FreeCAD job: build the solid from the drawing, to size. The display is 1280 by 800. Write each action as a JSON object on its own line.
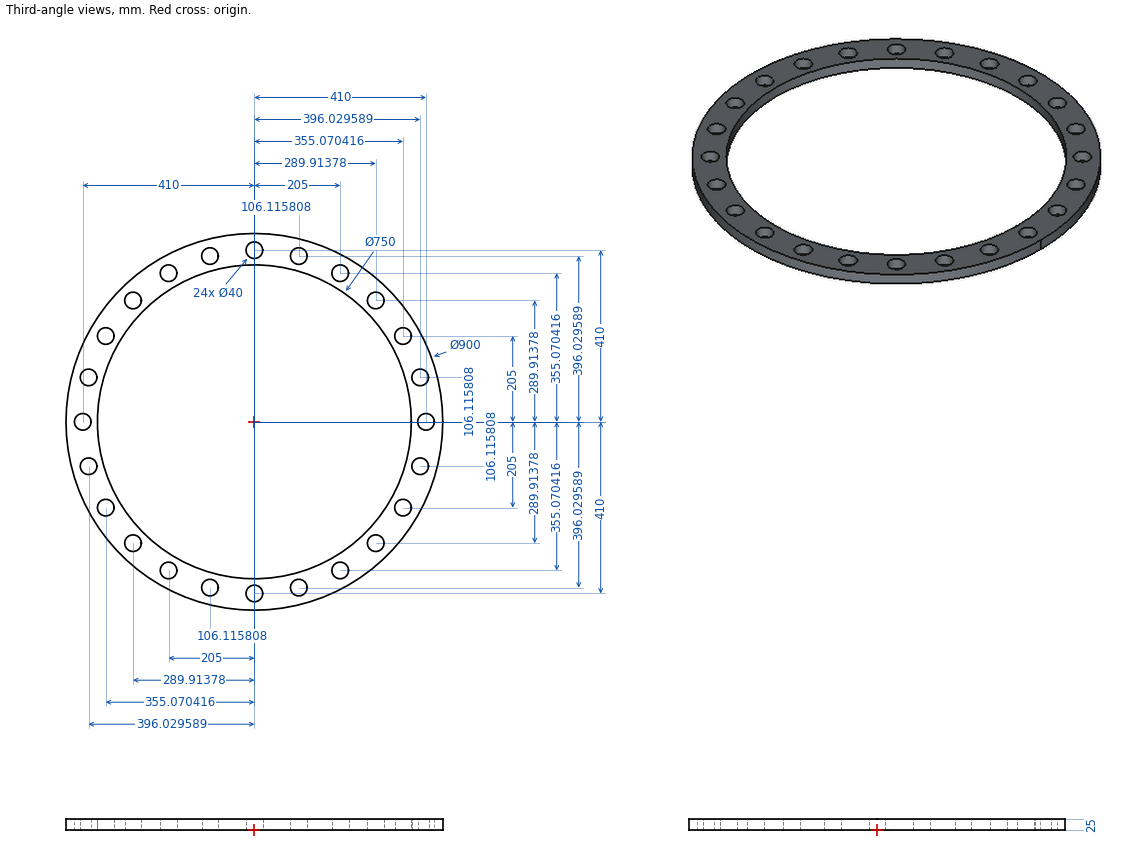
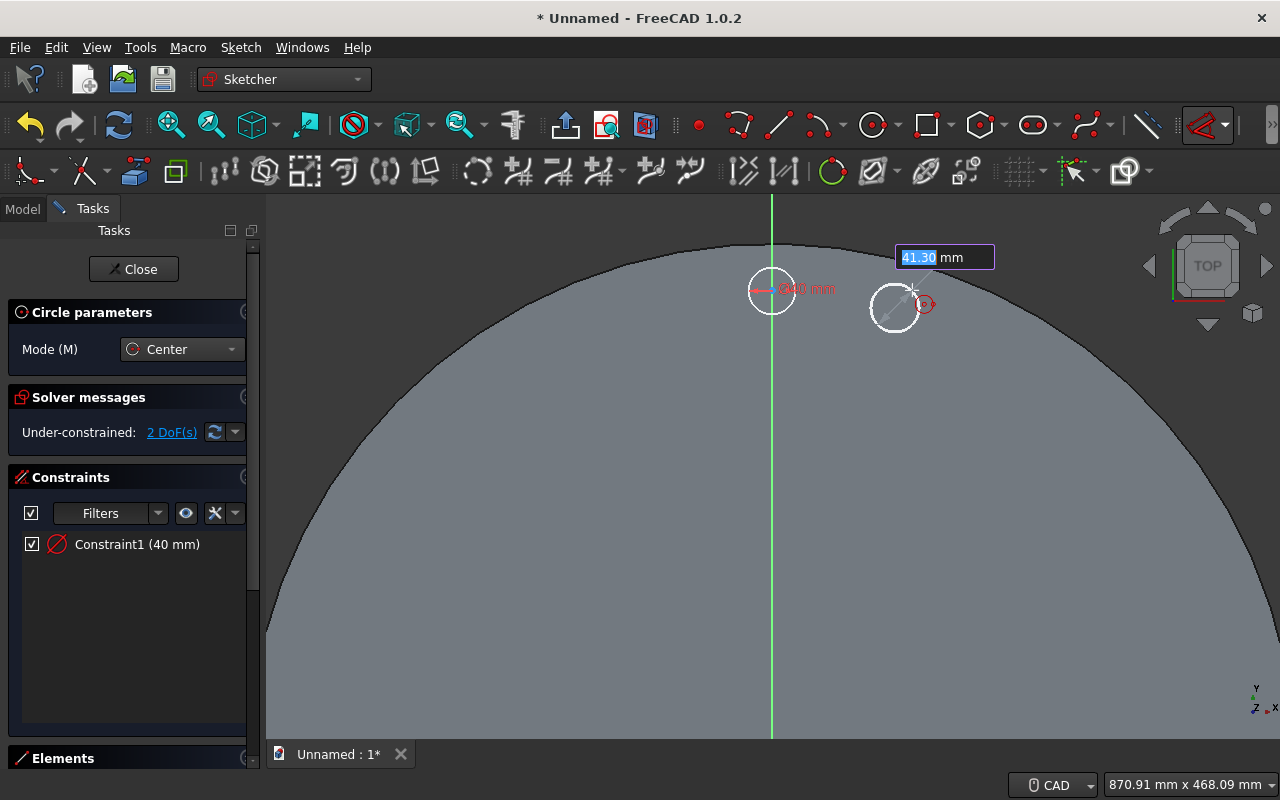
{"action": "type", "text": "40"}
{"action": "key", "text": "Return"}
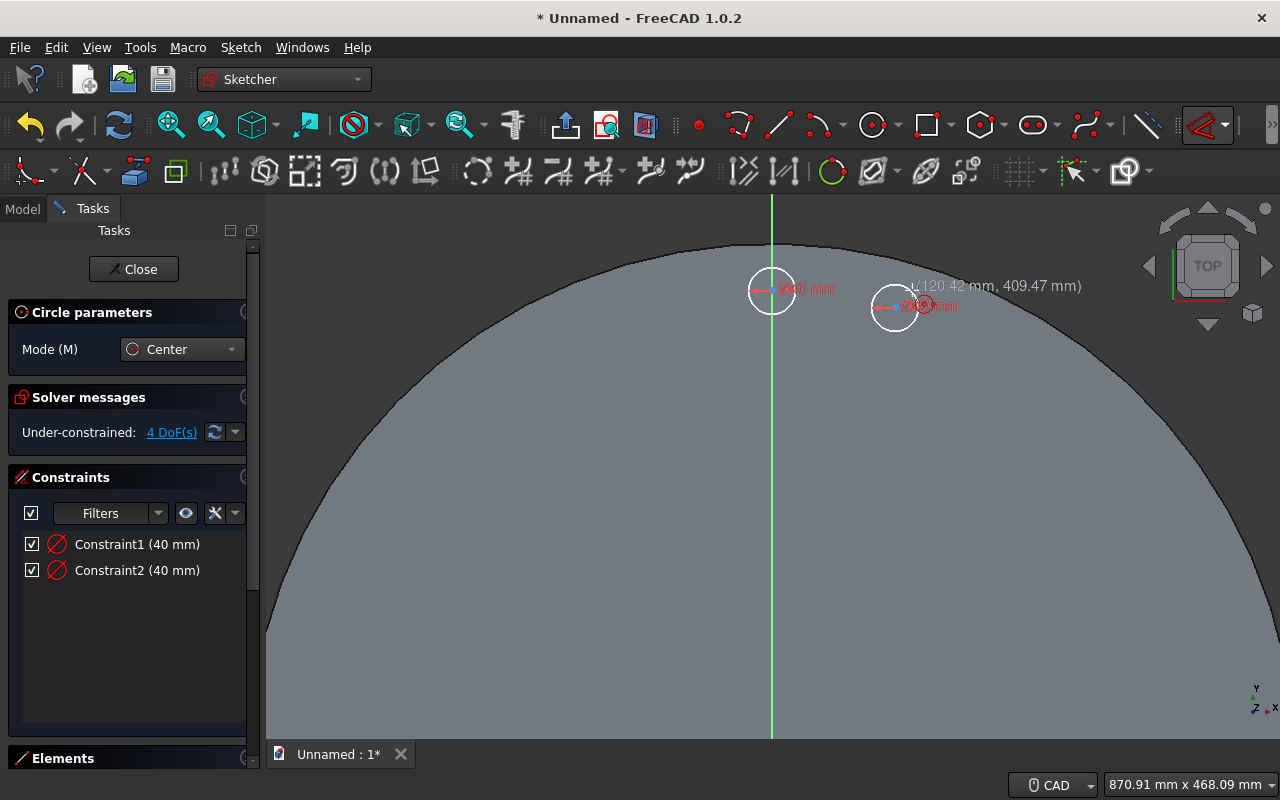
{"action": "left_click", "coordinate": [1010, 354]}
{"action": "mouse_move", "coordinate": [1027, 338]}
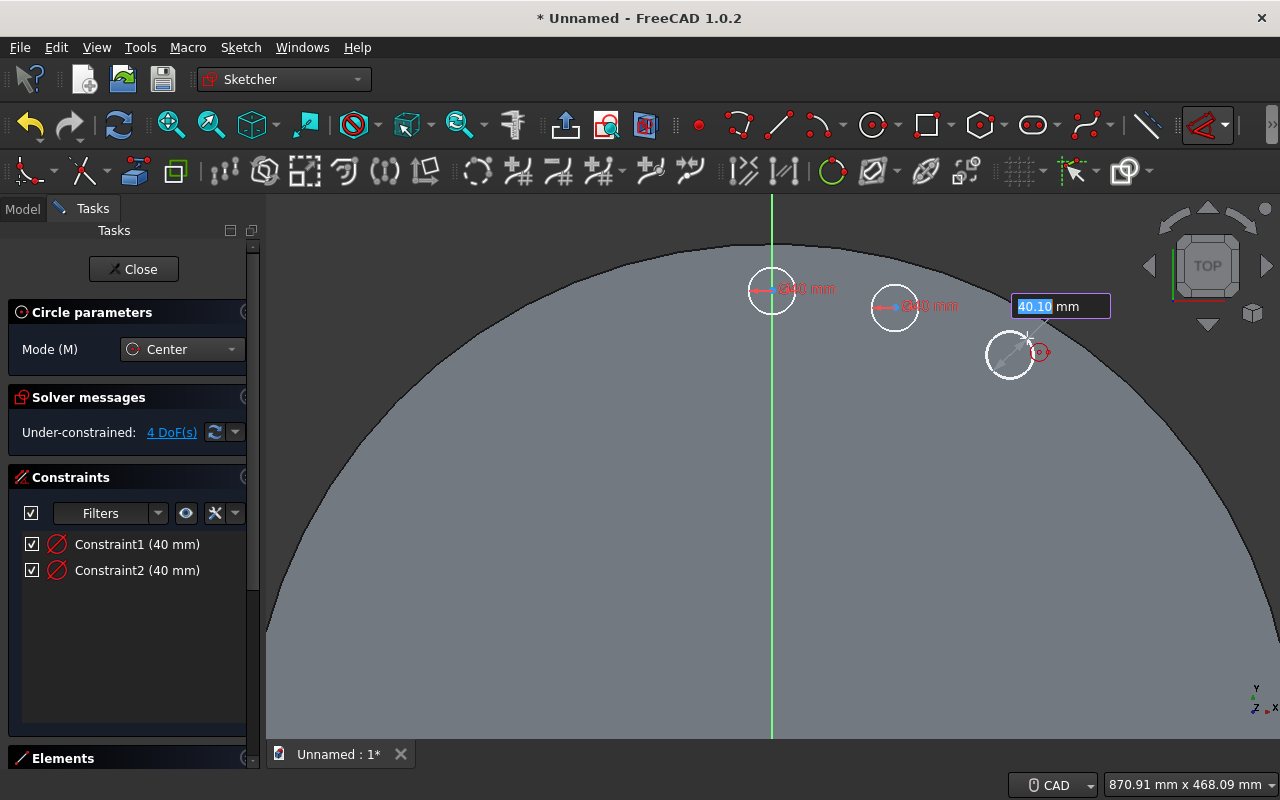
{"action": "type", "text": "40"}
{"action": "key", "text": "Return"}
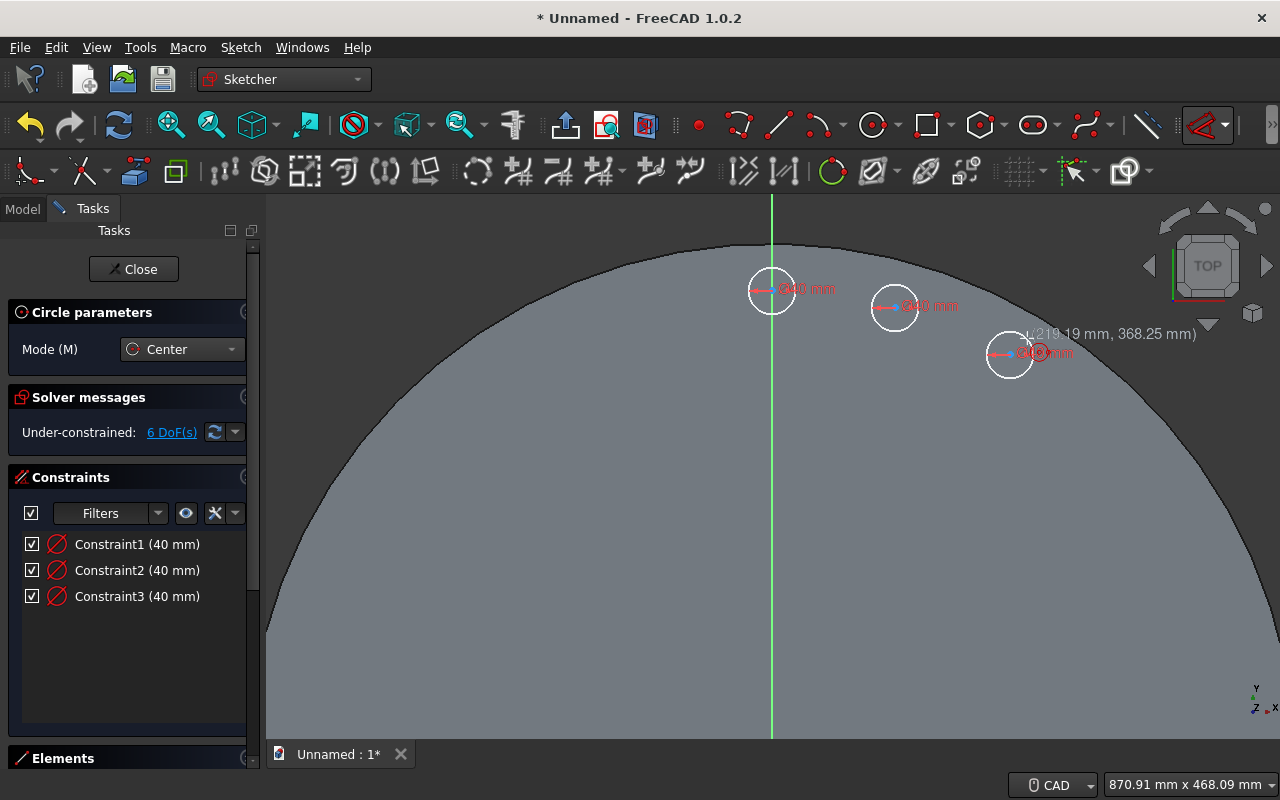
{"action": "left_click", "coordinate": [1109, 430]}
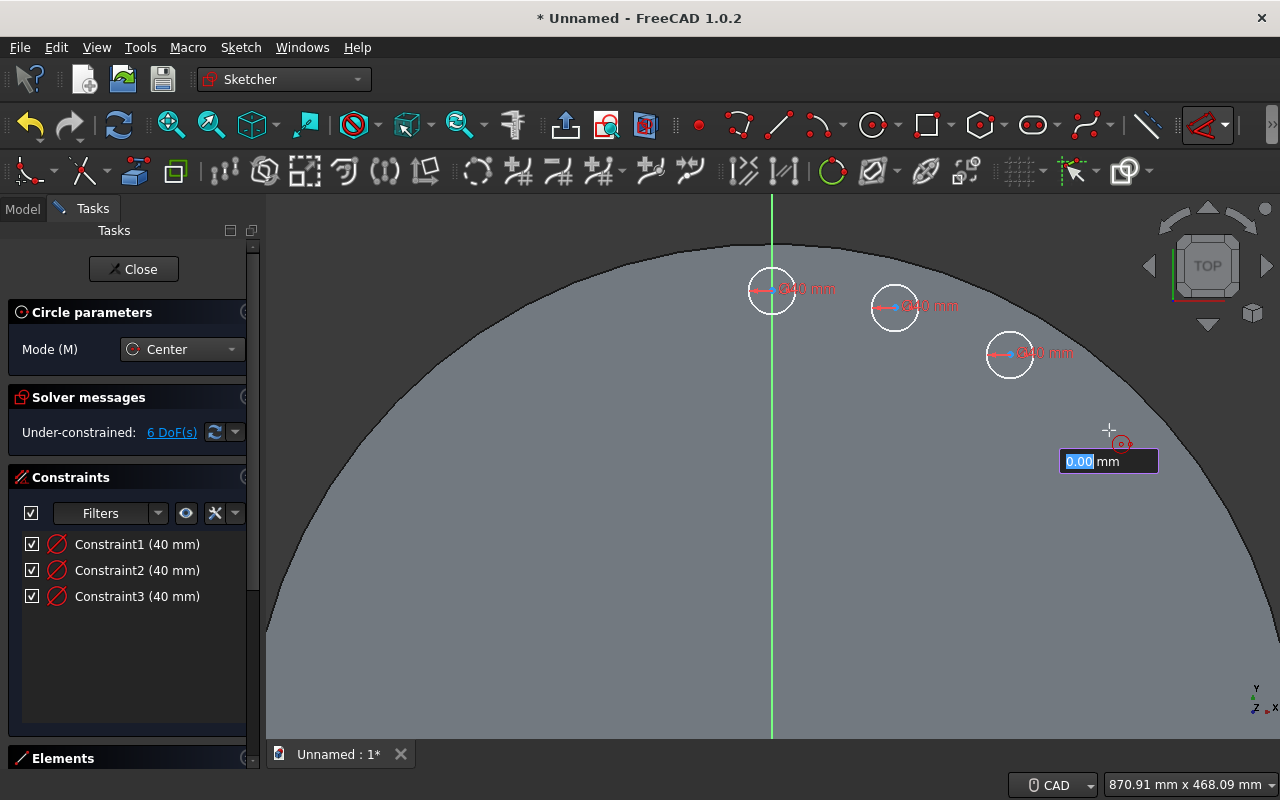
{"action": "scroll", "coordinate": [665, 291], "scroll_direction": "down", "scroll_amount": 5}
{"action": "mouse_move", "coordinate": [835, 336]}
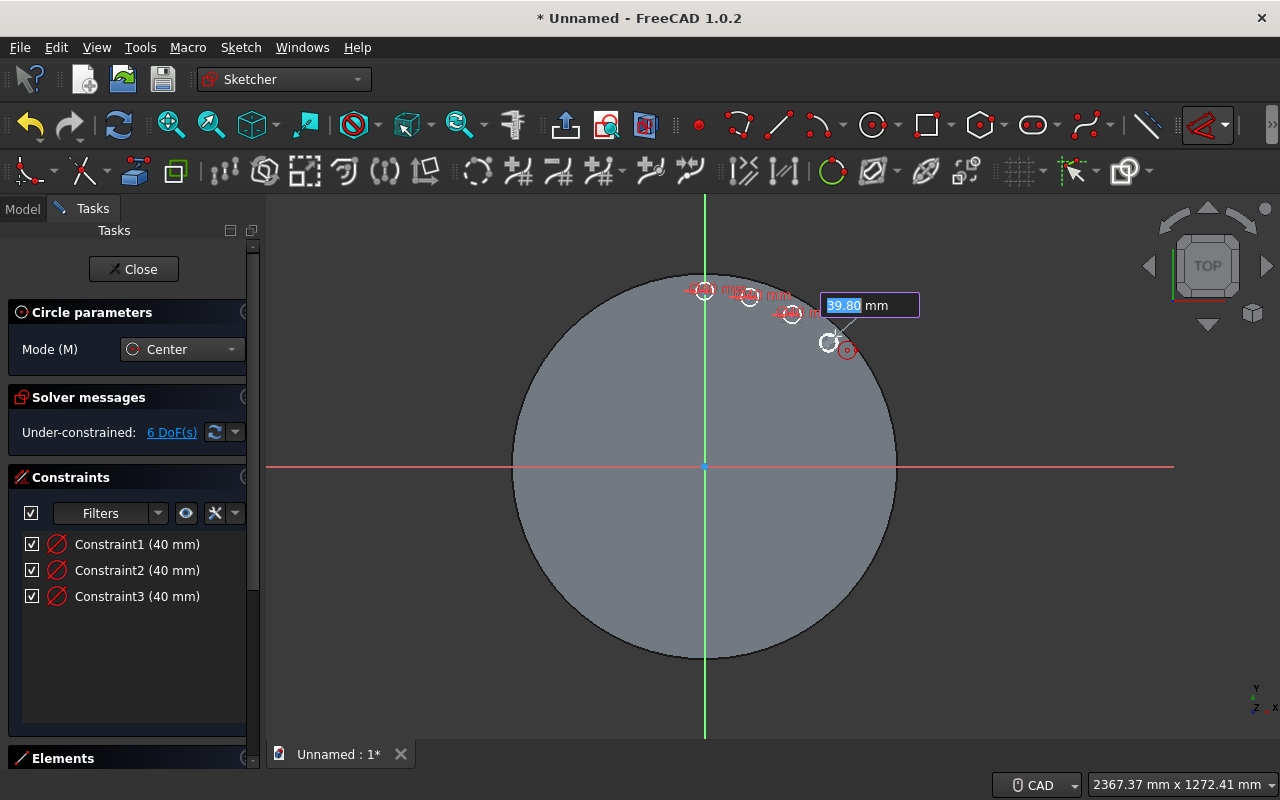
{"action": "type", "text": "40"}
{"action": "key", "text": "Return"}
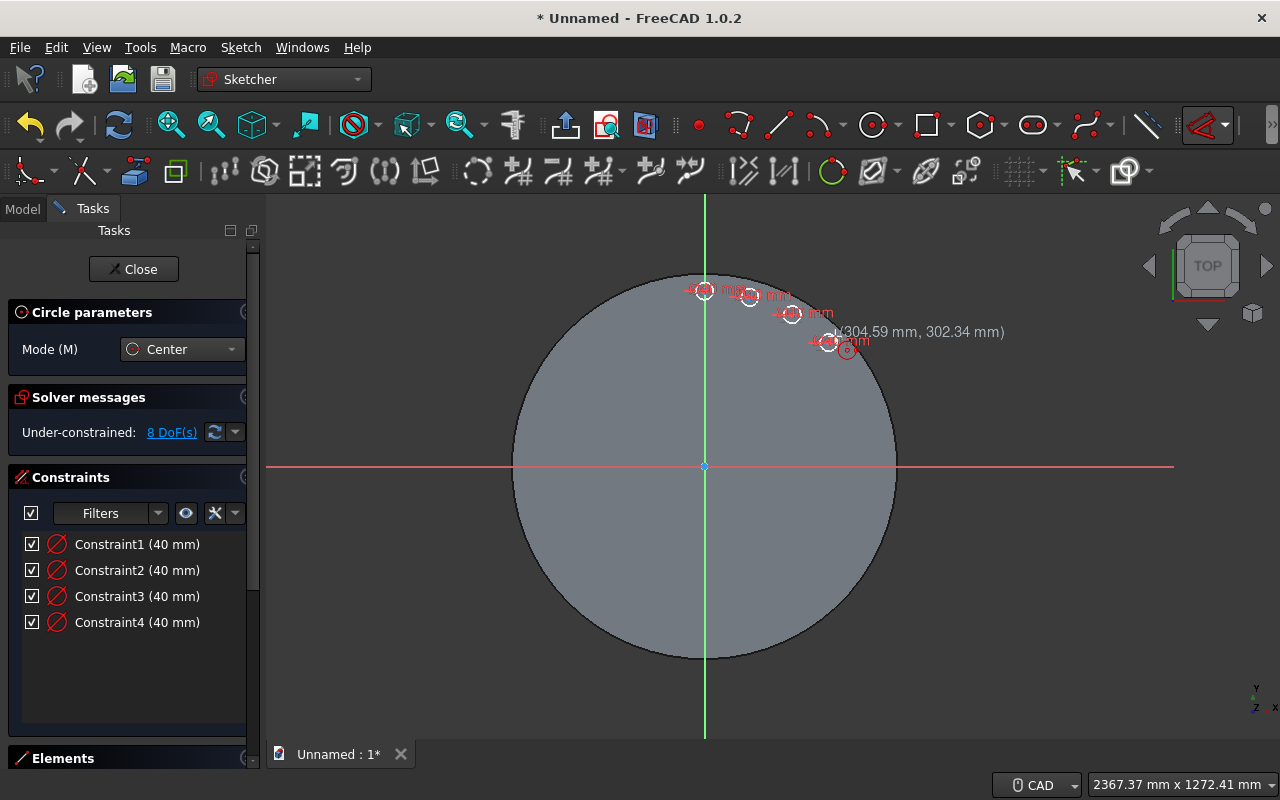
{"action": "scroll", "coordinate": [857, 379], "scroll_direction": "up", "scroll_amount": 5}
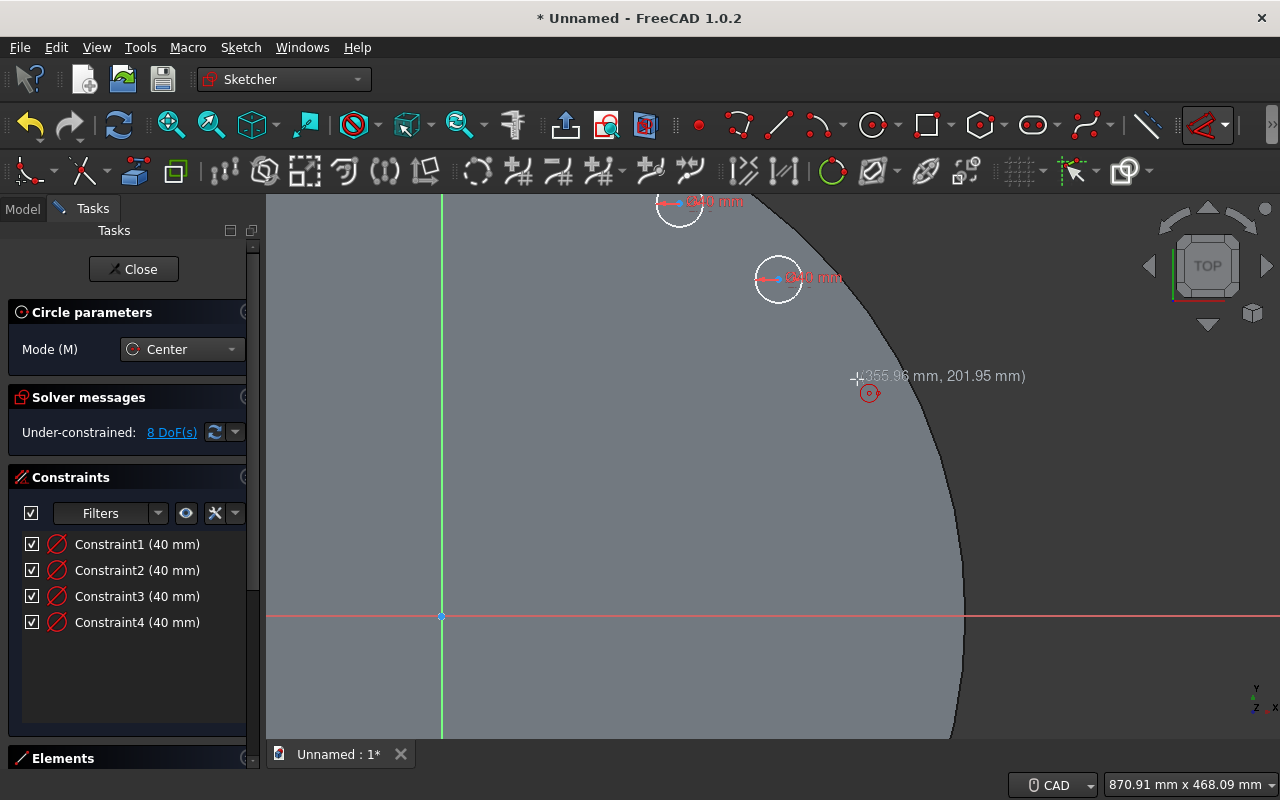
{"action": "left_click", "coordinate": [855, 378]}
{"action": "mouse_move", "coordinate": [871, 361]}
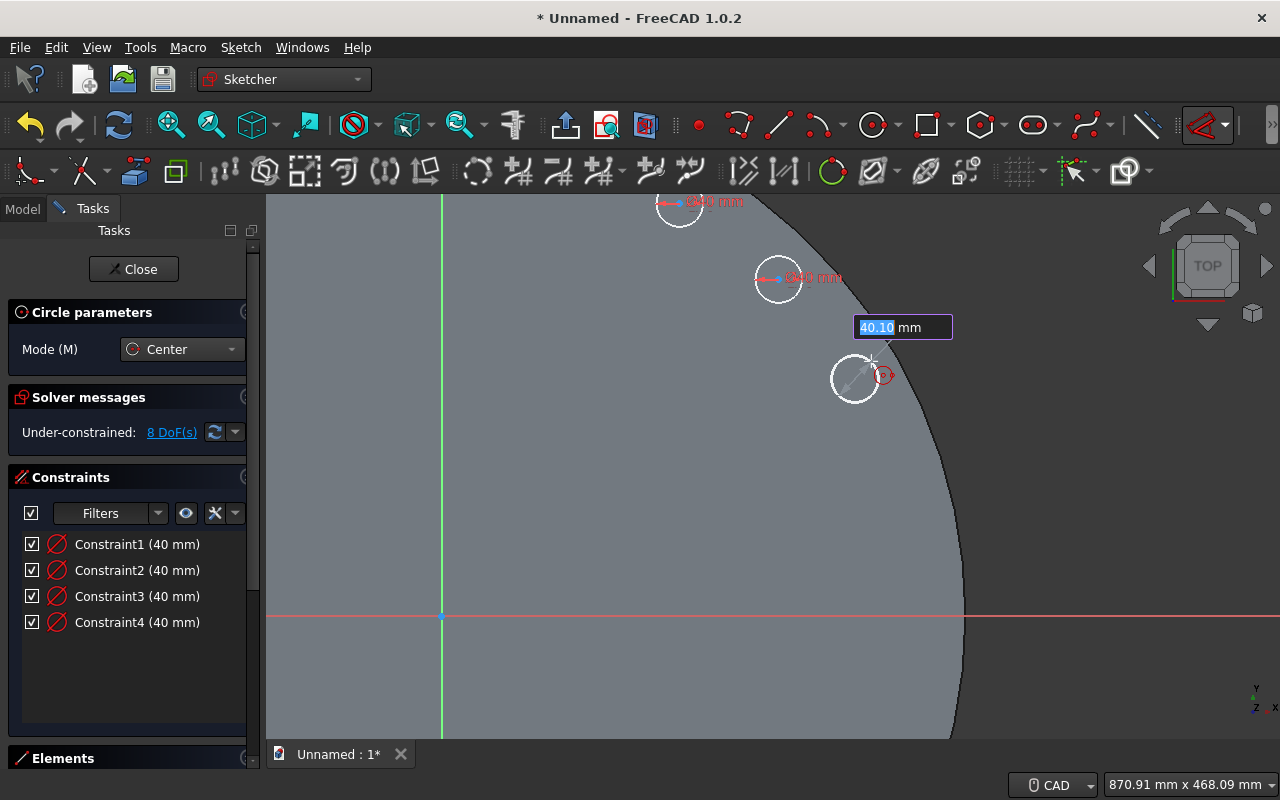
{"action": "type", "text": "40"}
{"action": "key", "text": "Return"}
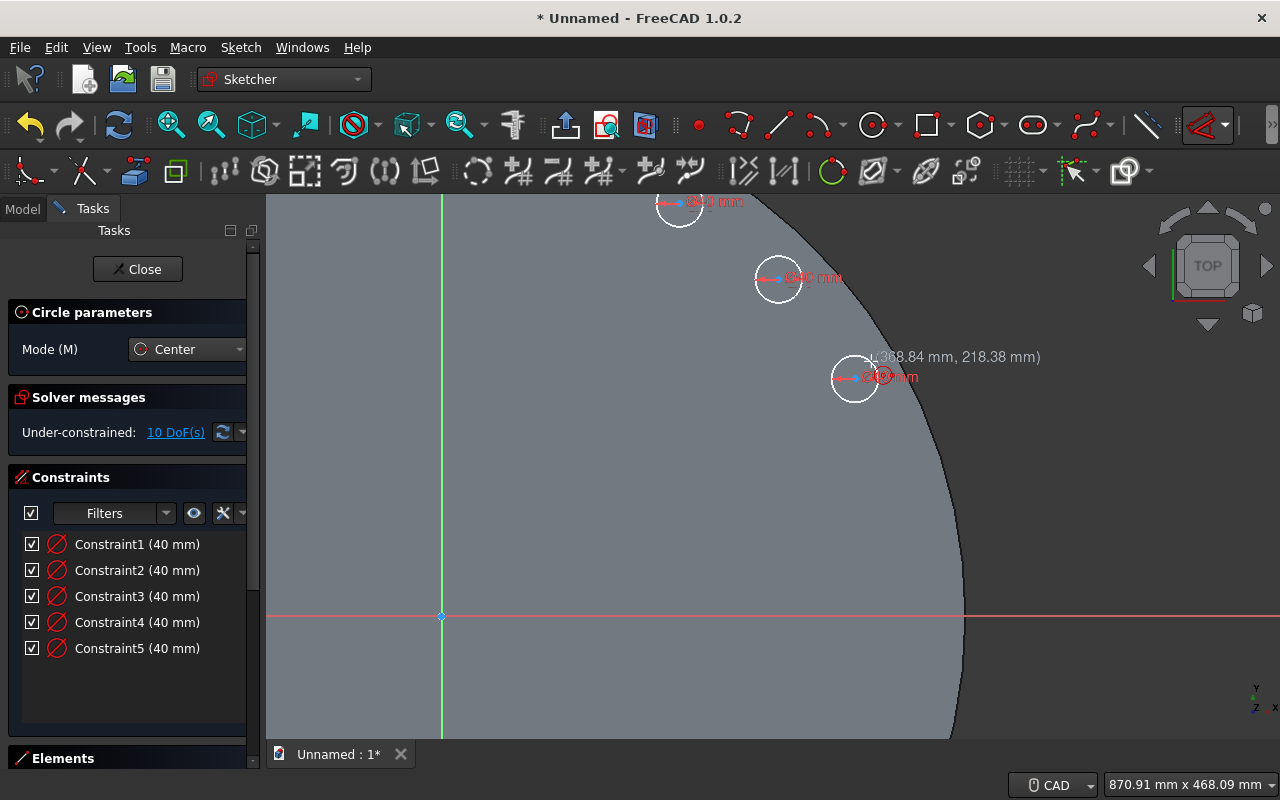
{"action": "left_click", "coordinate": [903, 493]}
{"action": "mouse_move", "coordinate": [919, 476]}